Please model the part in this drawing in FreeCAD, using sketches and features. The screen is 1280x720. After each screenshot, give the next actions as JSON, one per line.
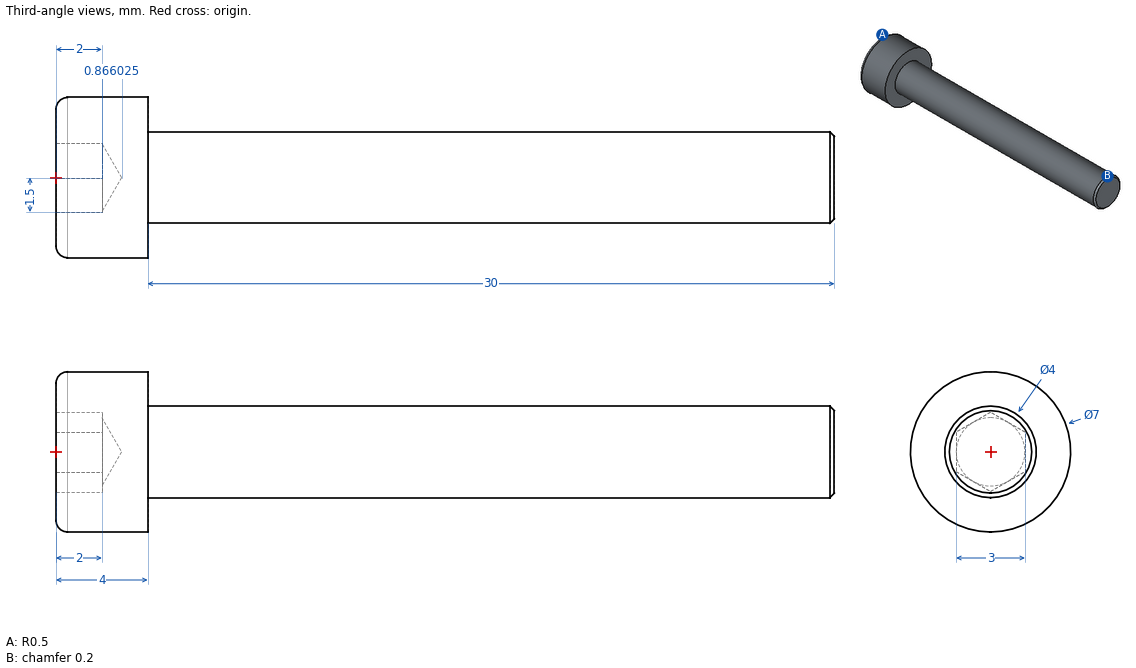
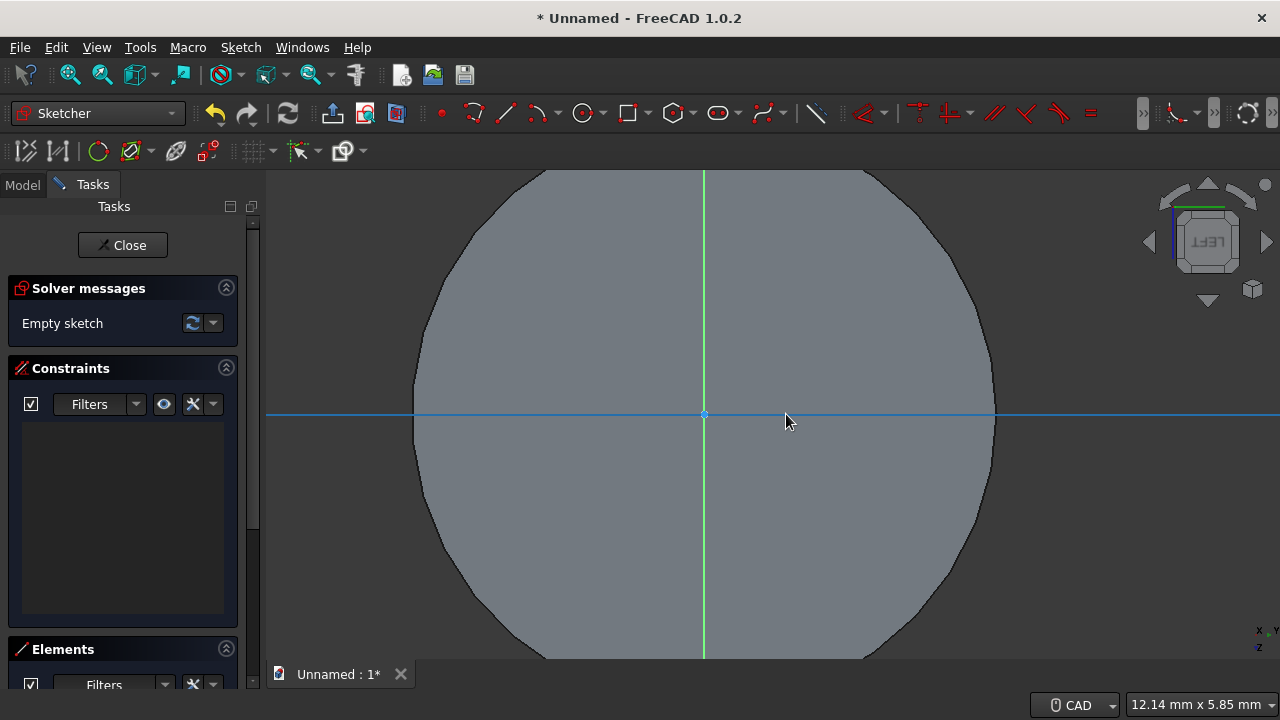
{"action": "left_click", "coordinate": [674, 114]}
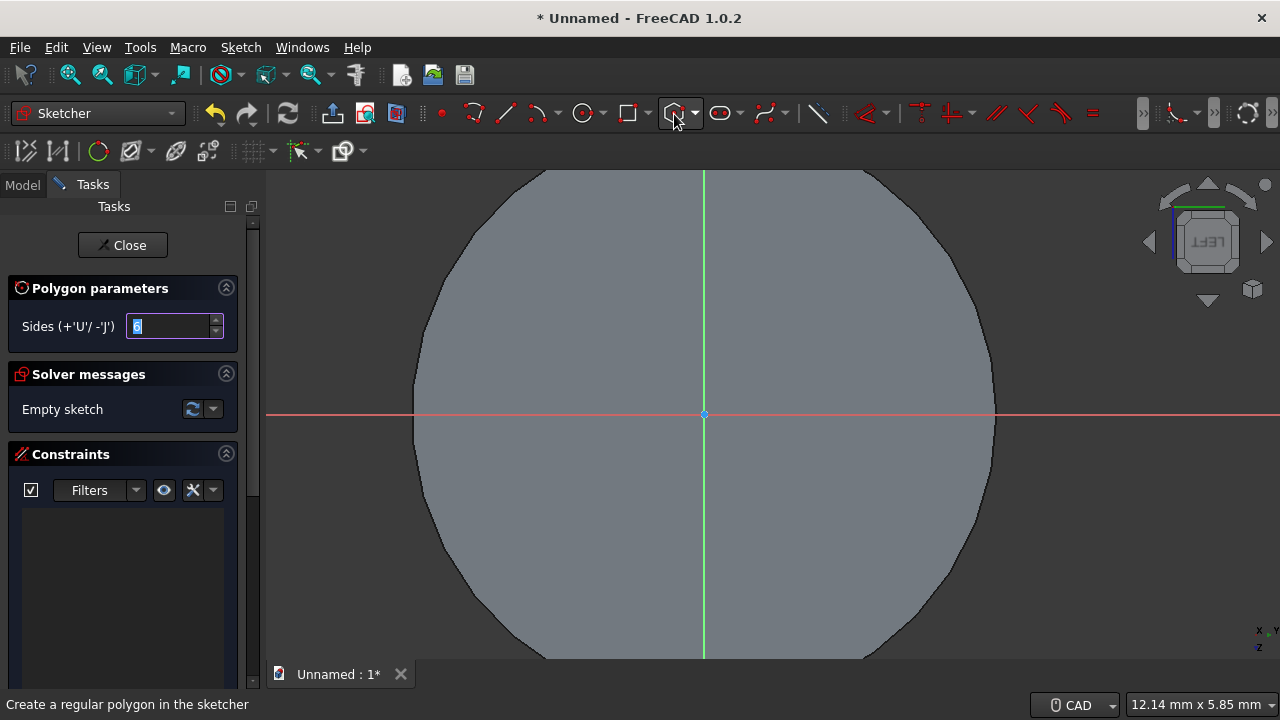
{"action": "left_click", "coordinate": [704, 414]}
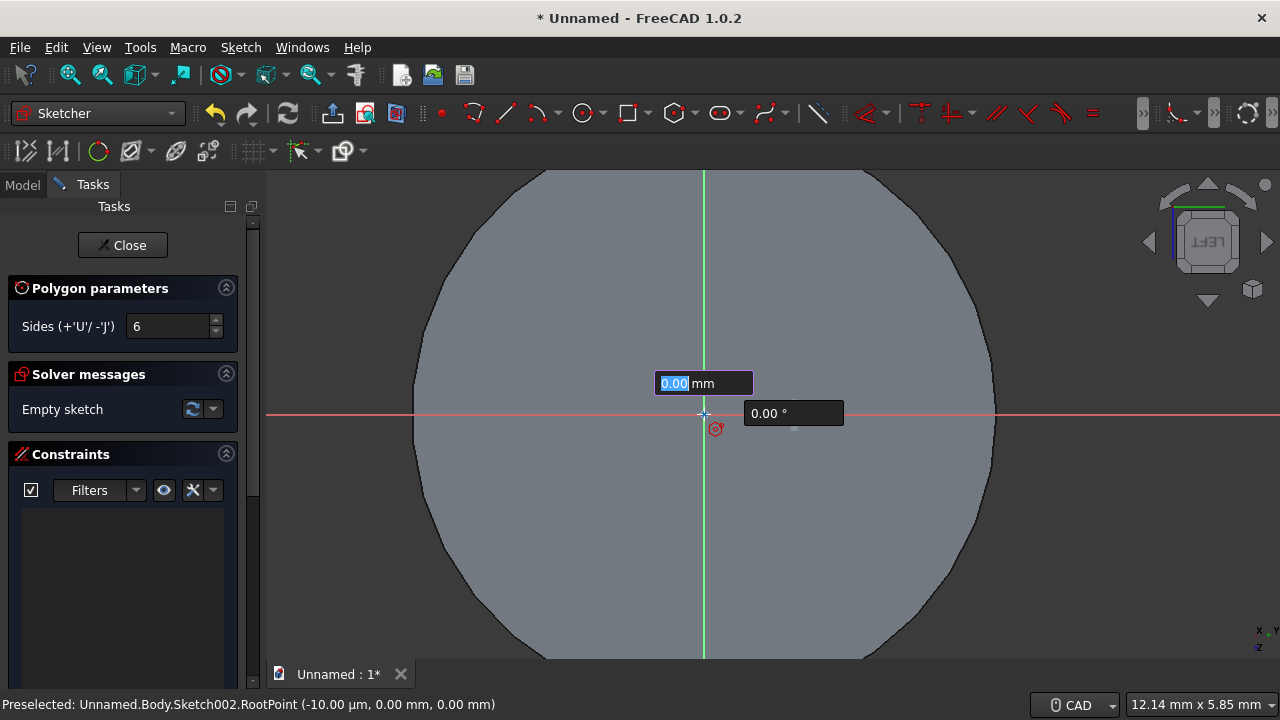
{"action": "left_click", "coordinate": [704, 270]}
{"action": "key", "text": "Escape"}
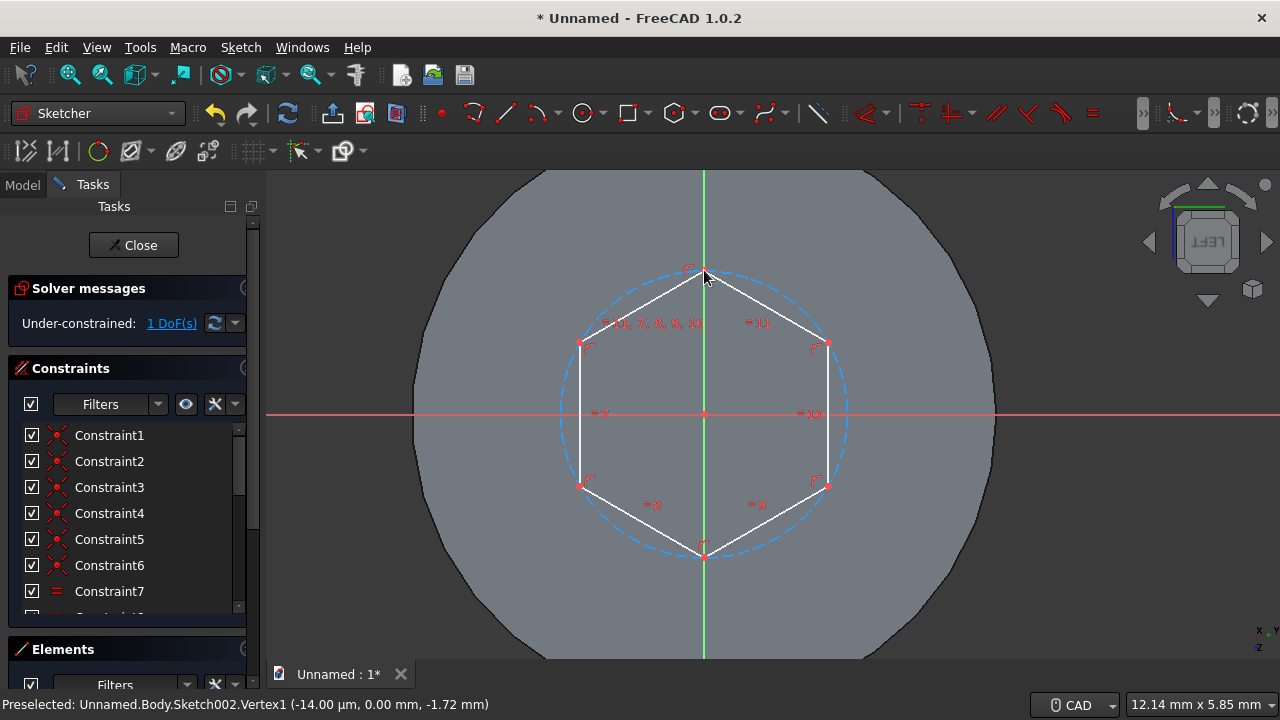
{"action": "left_click", "coordinate": [866, 114]}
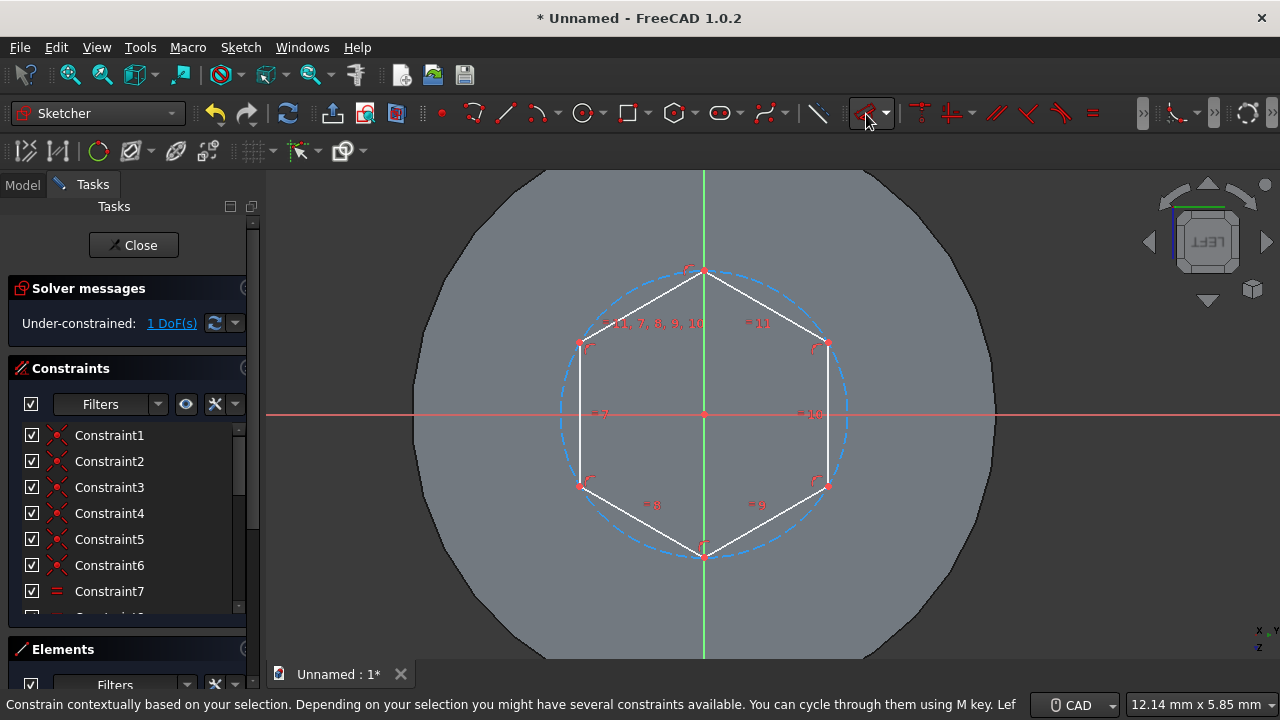
{"action": "left_click", "coordinate": [580, 343]}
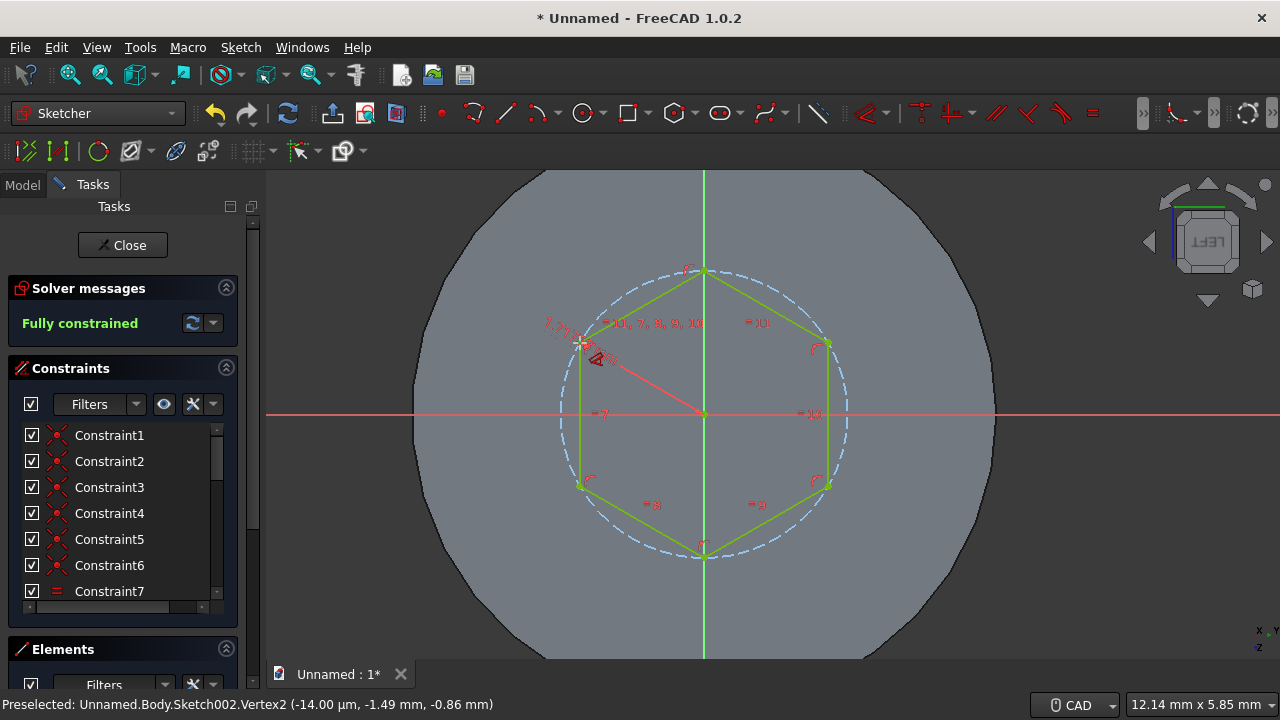
{"action": "left_click", "coordinate": [828, 486]}
{"action": "left_click", "coordinate": [647, 568]}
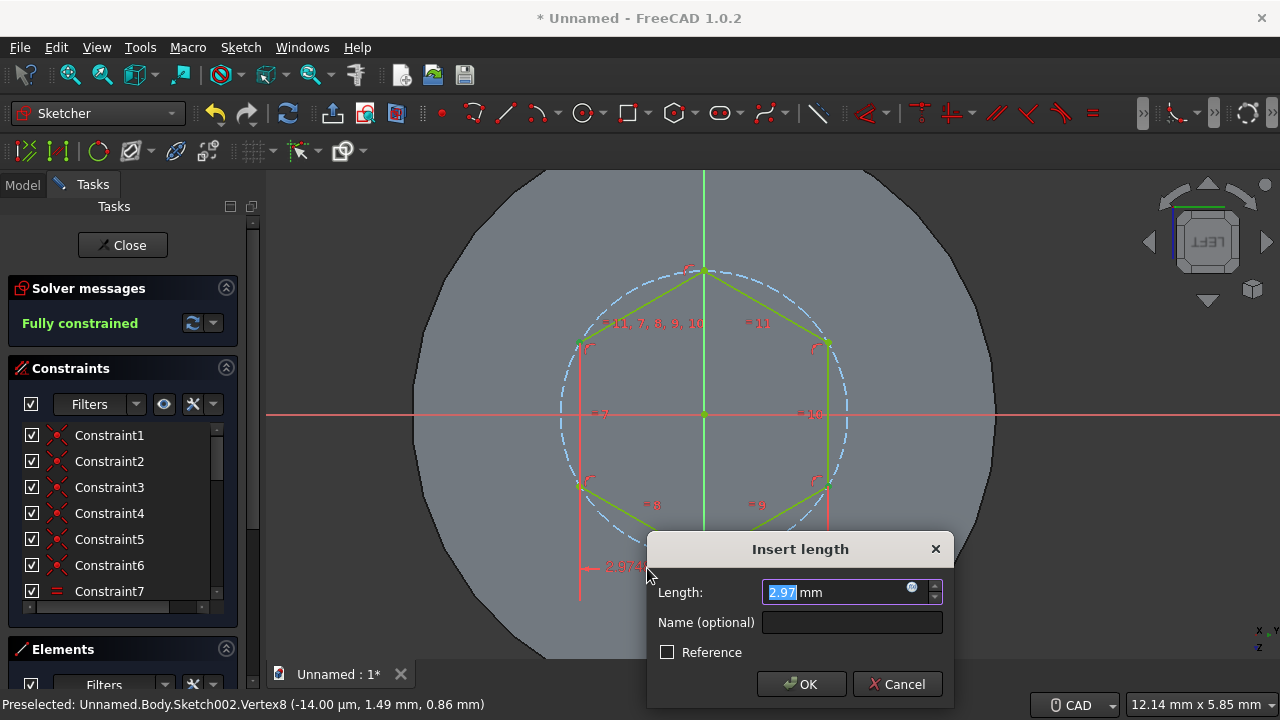
{"action": "type", "text": "3"}
{"action": "key", "text": "Return"}
{"action": "key", "text": "Escape"}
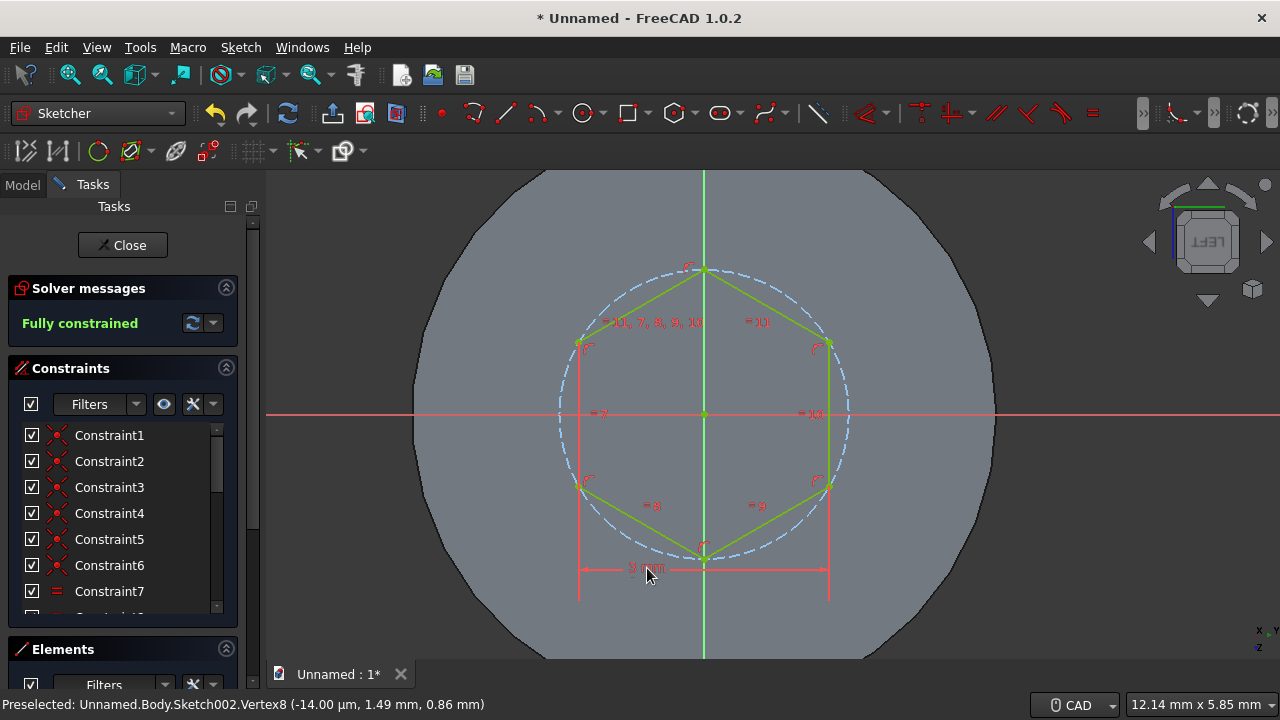
{"action": "left_click", "coordinate": [123, 245]}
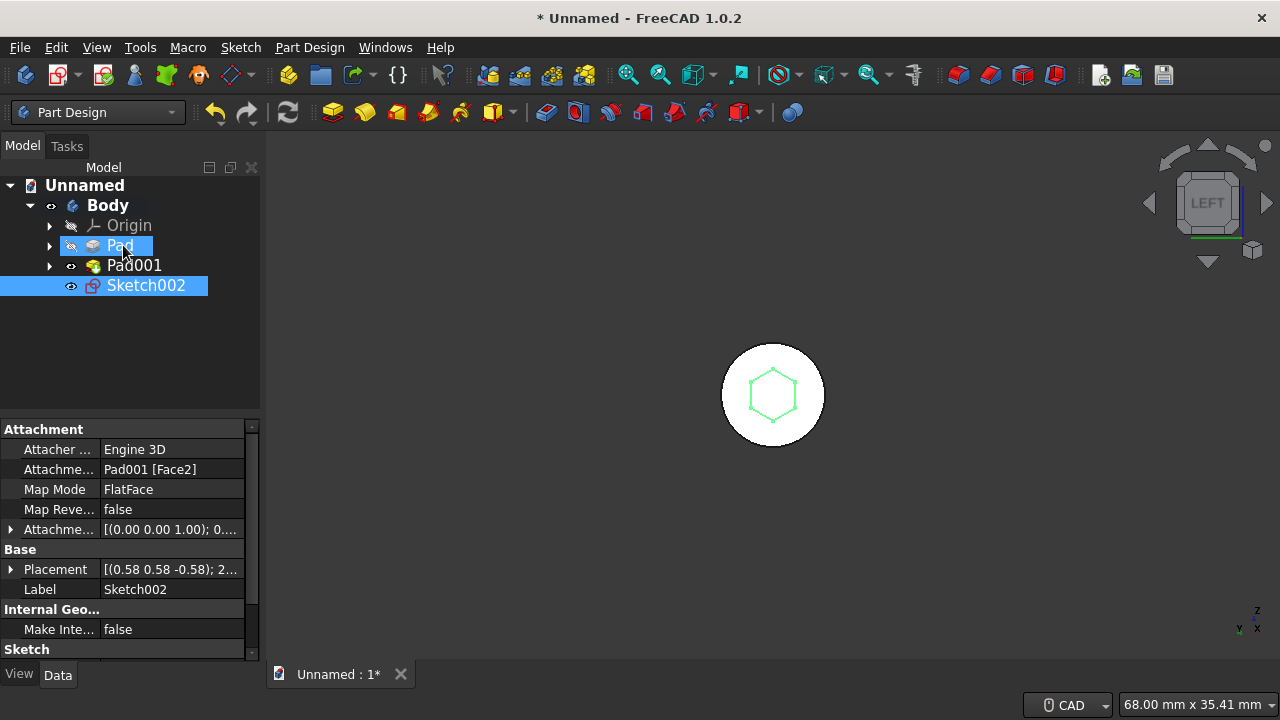
{"action": "left_click", "coordinate": [548, 112]}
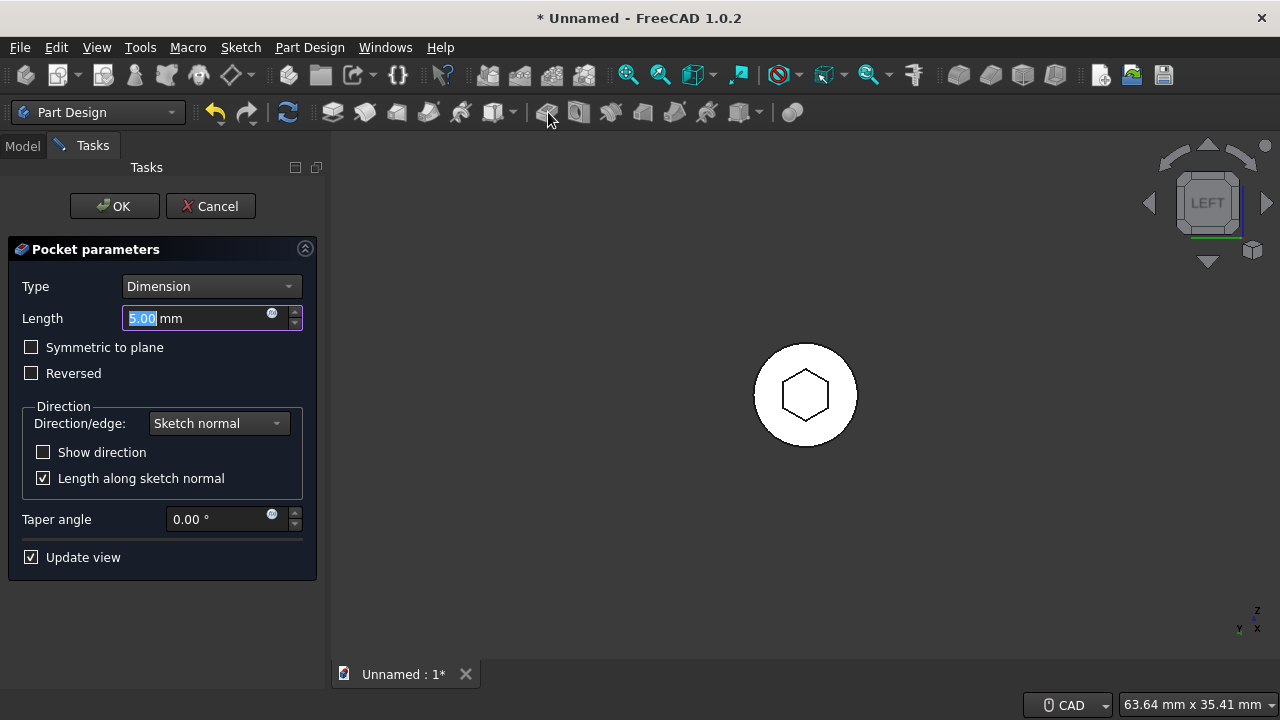
{"action": "type", "text": "2"}
{"action": "key", "text": "Tab"}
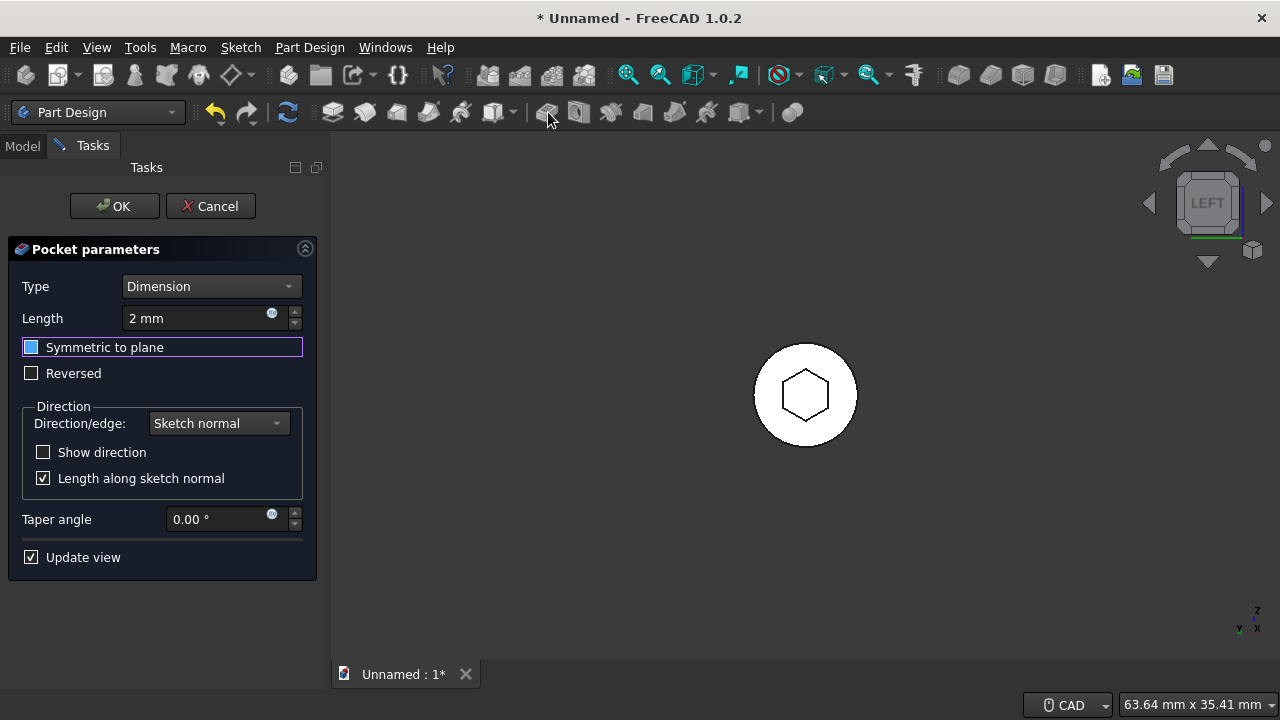
{"action": "left_click", "coordinate": [115, 206]}